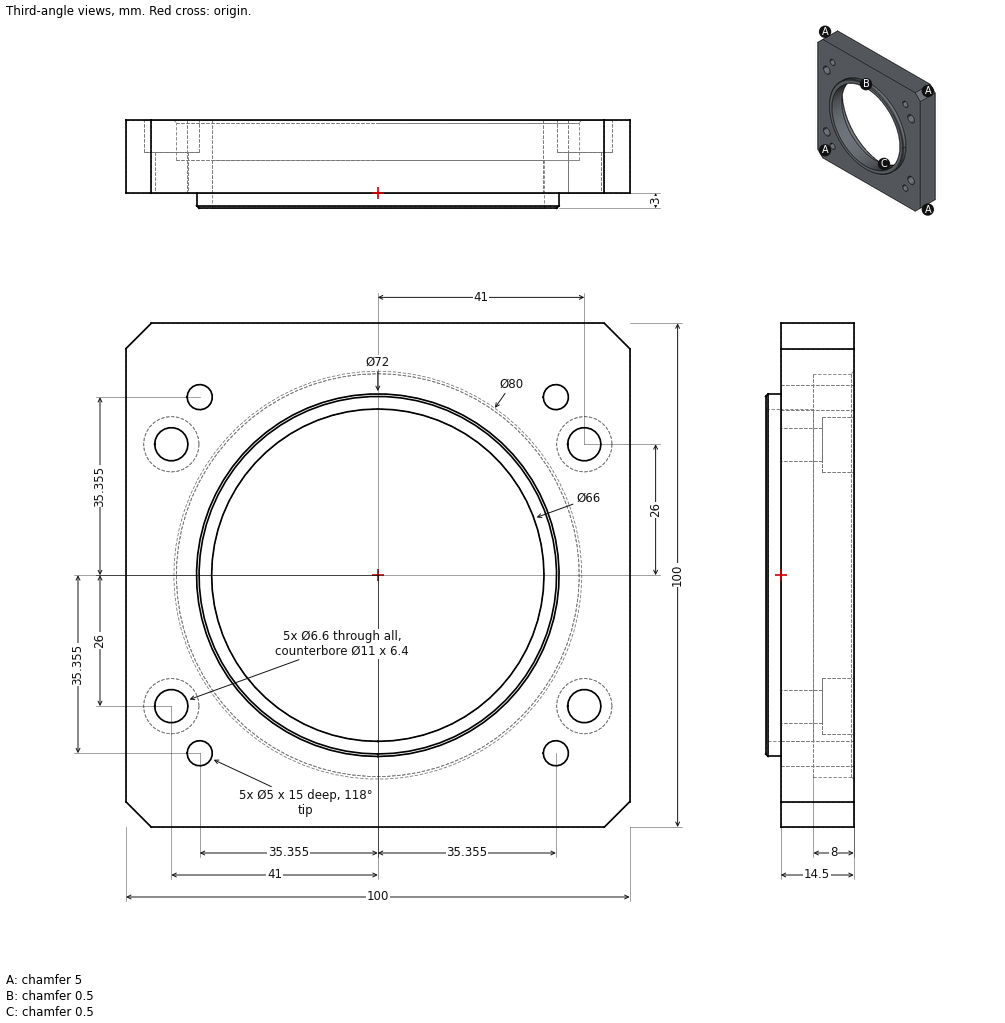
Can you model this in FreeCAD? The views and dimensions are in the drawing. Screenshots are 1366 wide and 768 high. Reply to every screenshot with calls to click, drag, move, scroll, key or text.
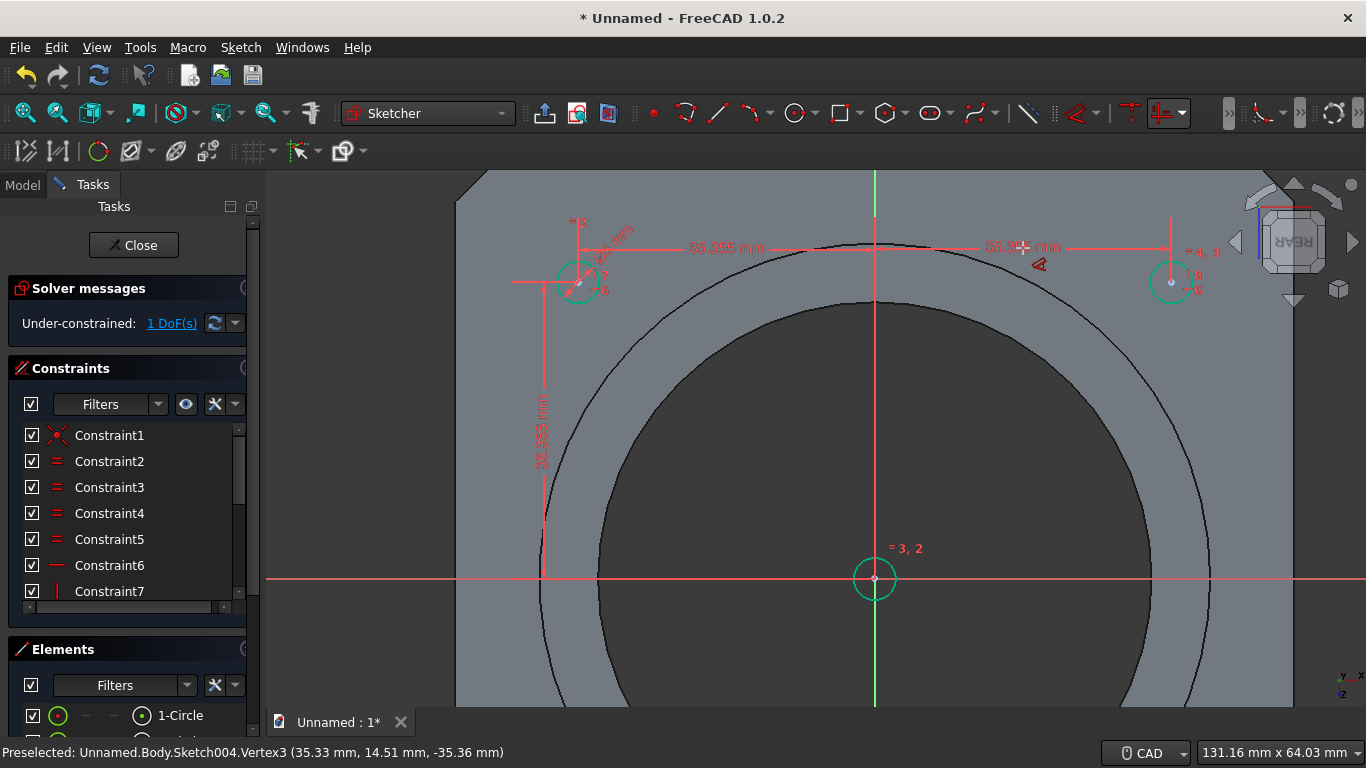
scroll(593, 268, down, 3)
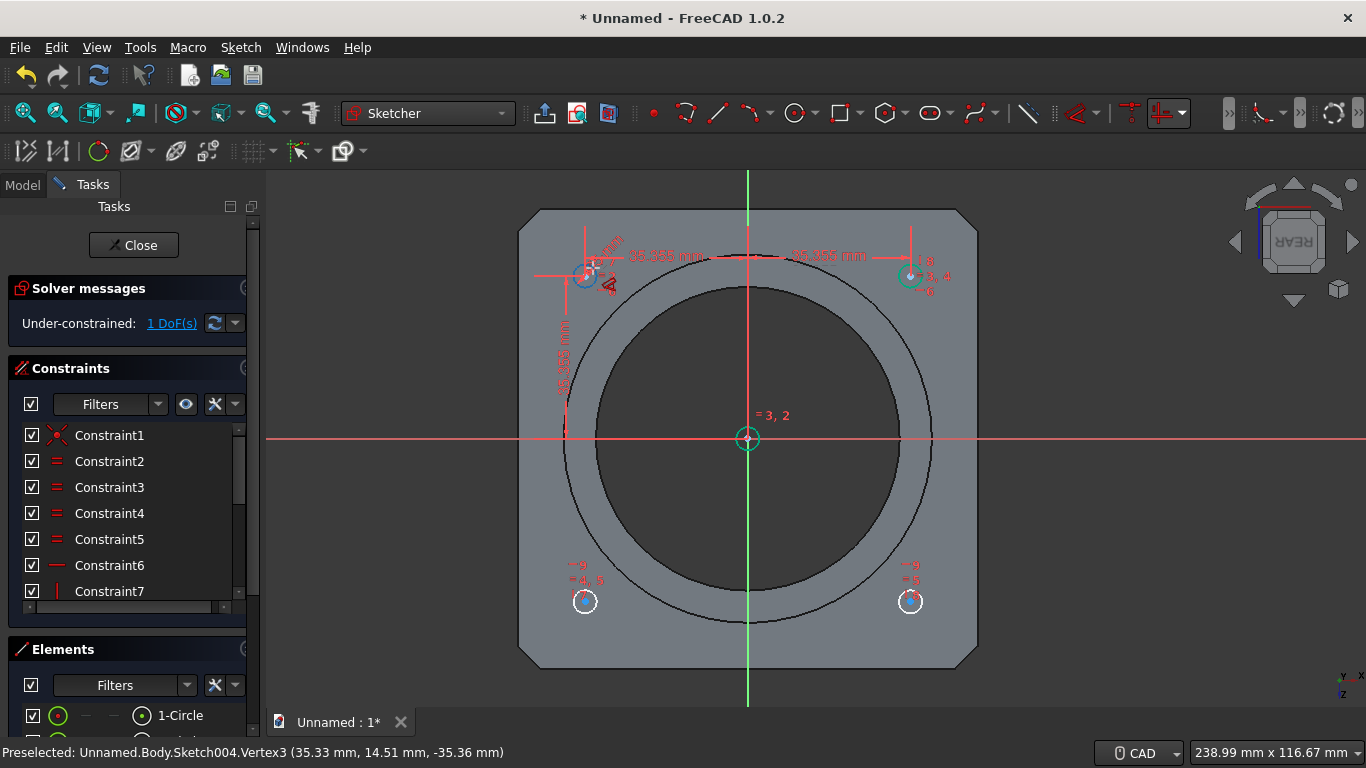
click(585, 602)
click(551, 520)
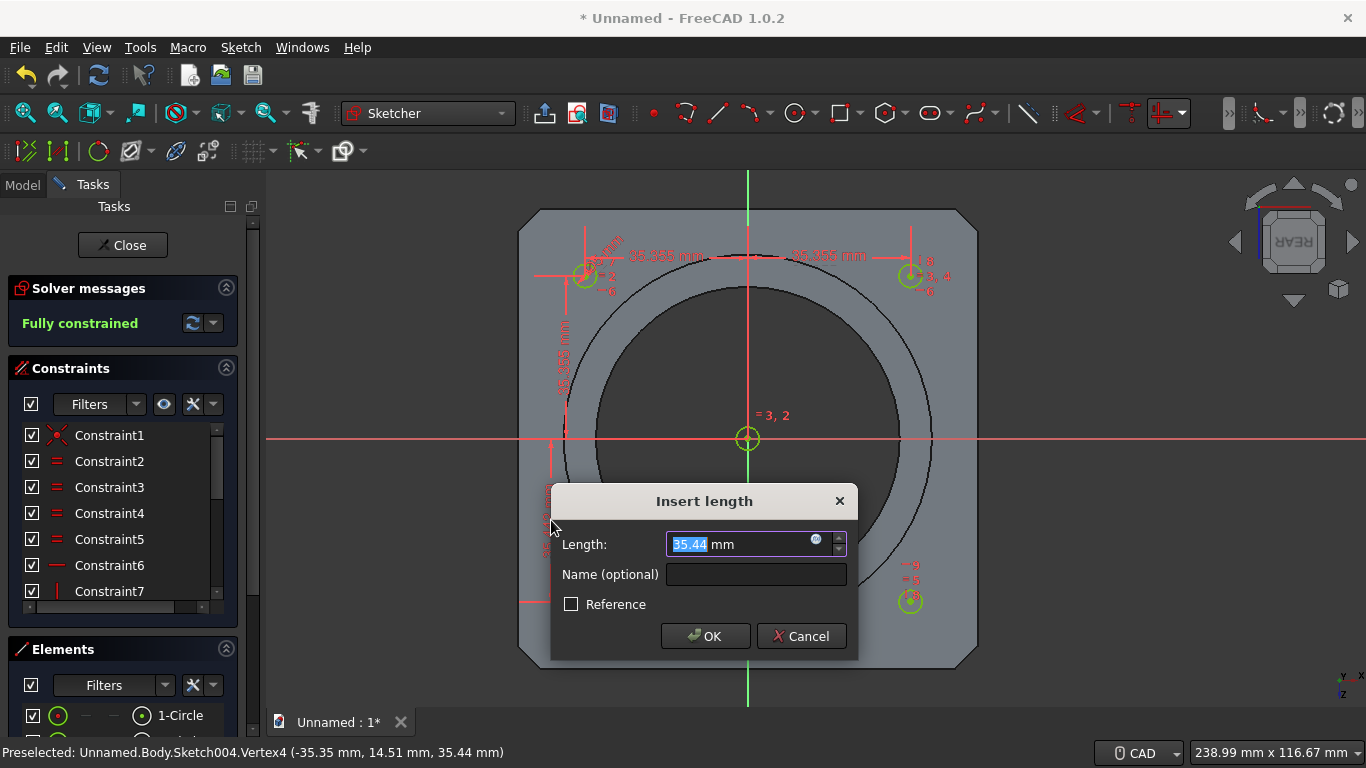
text(35.355)
key(Return)
key(Escape)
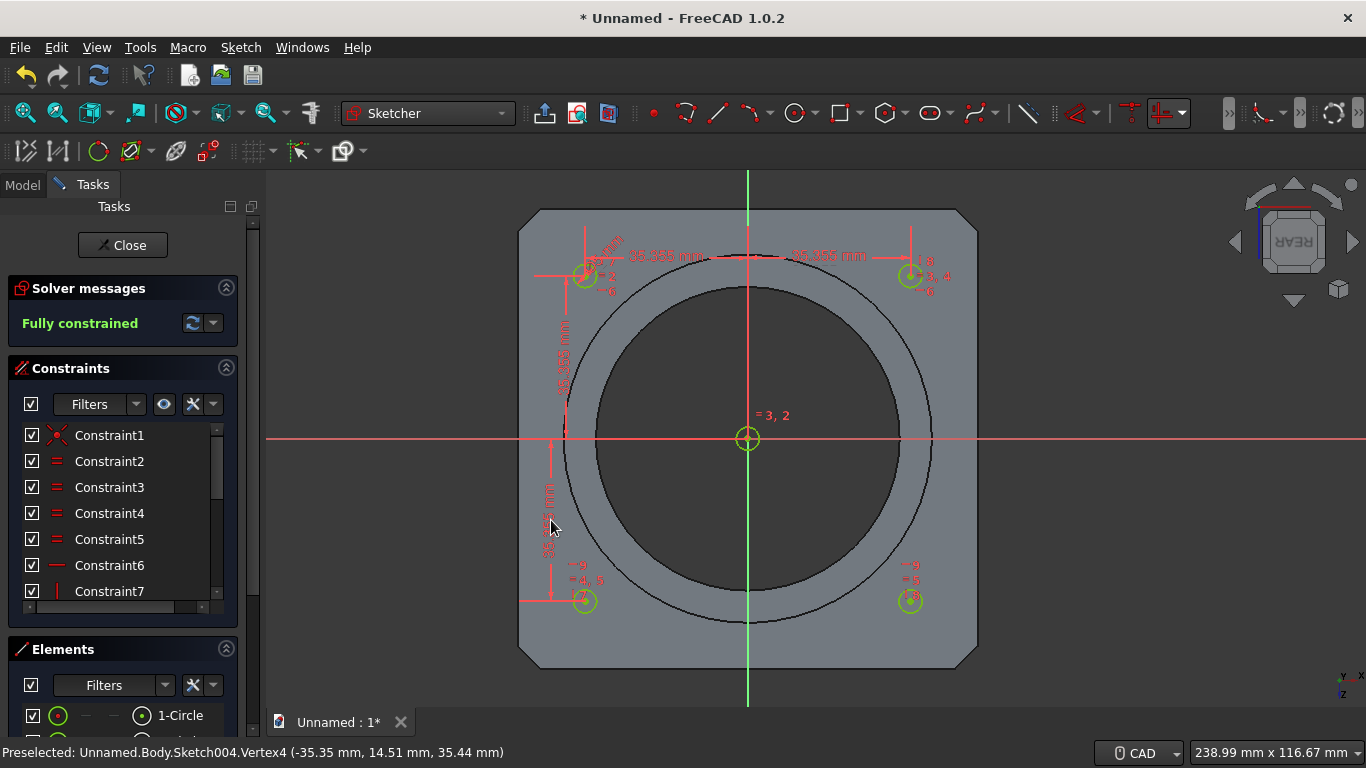
click(123, 245)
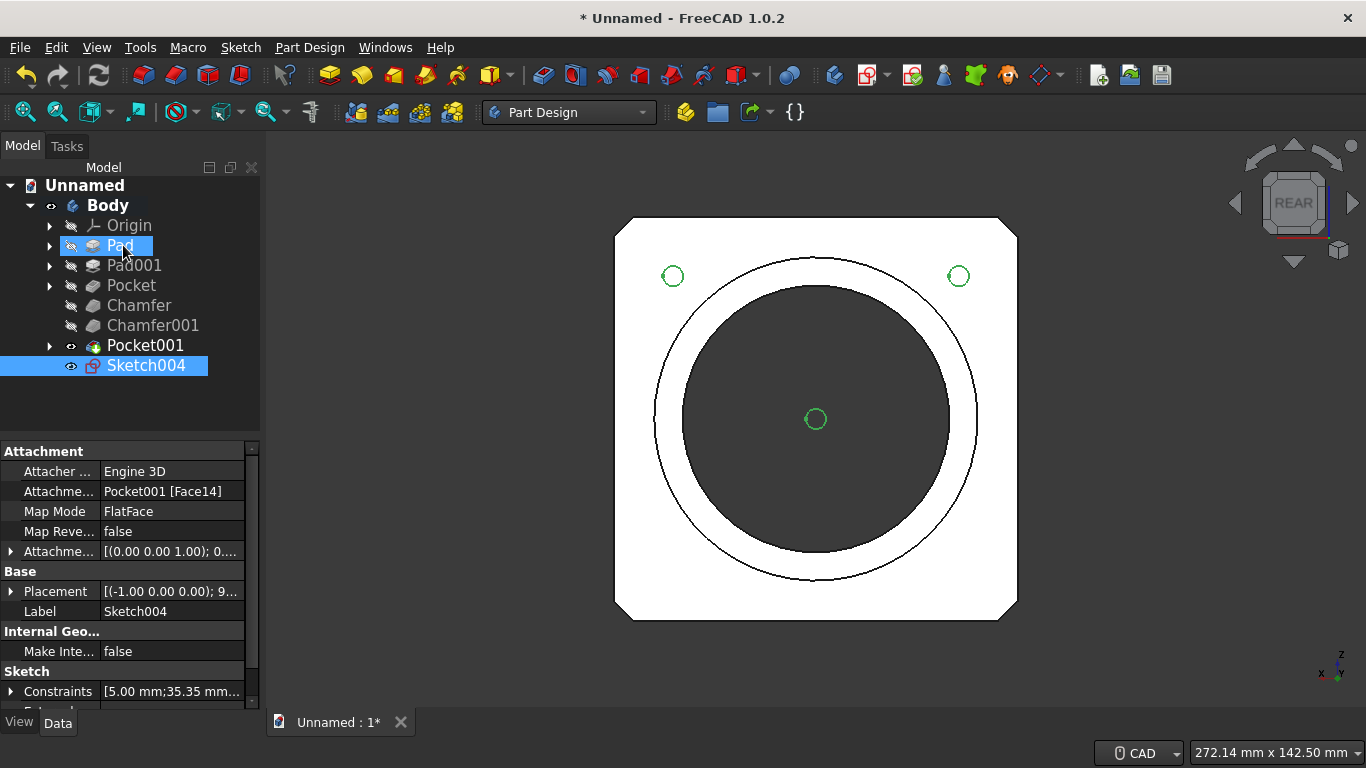
click(576, 76)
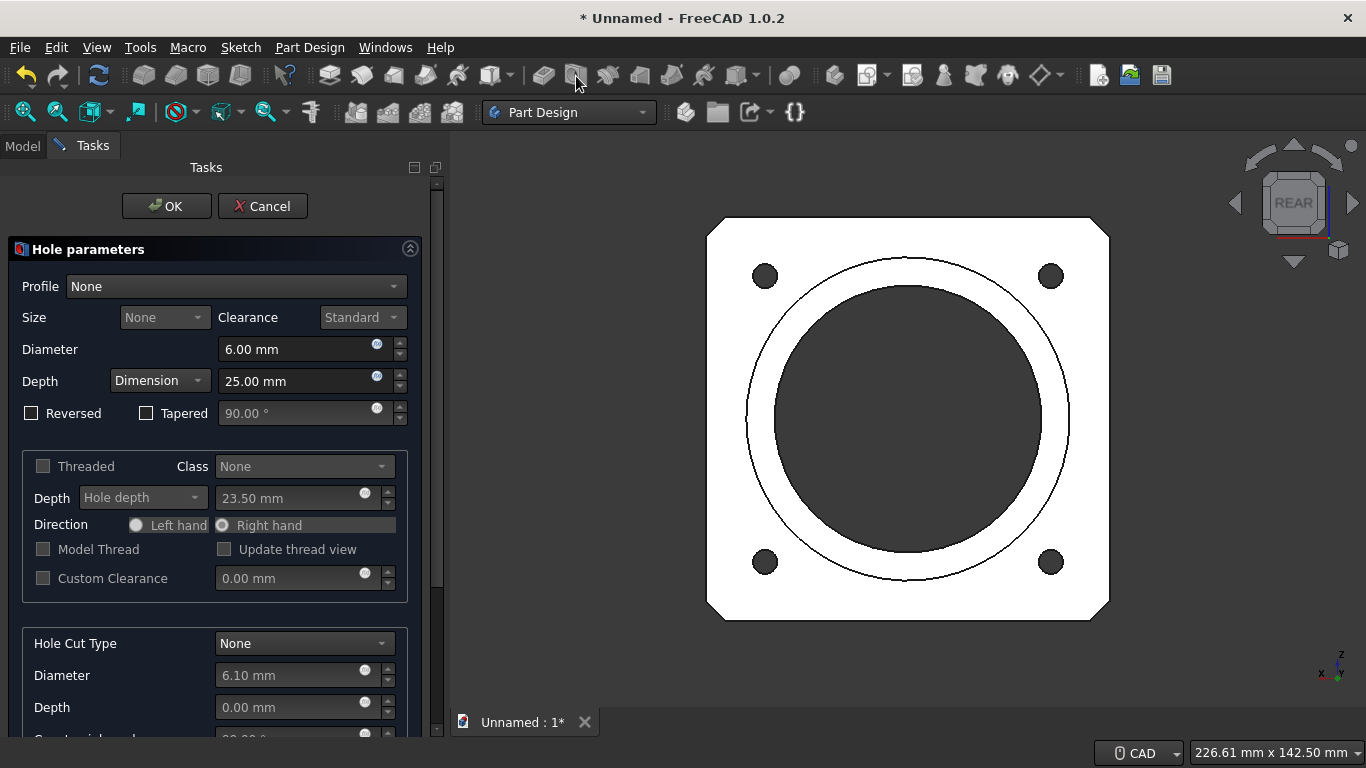
triple_click(305, 349)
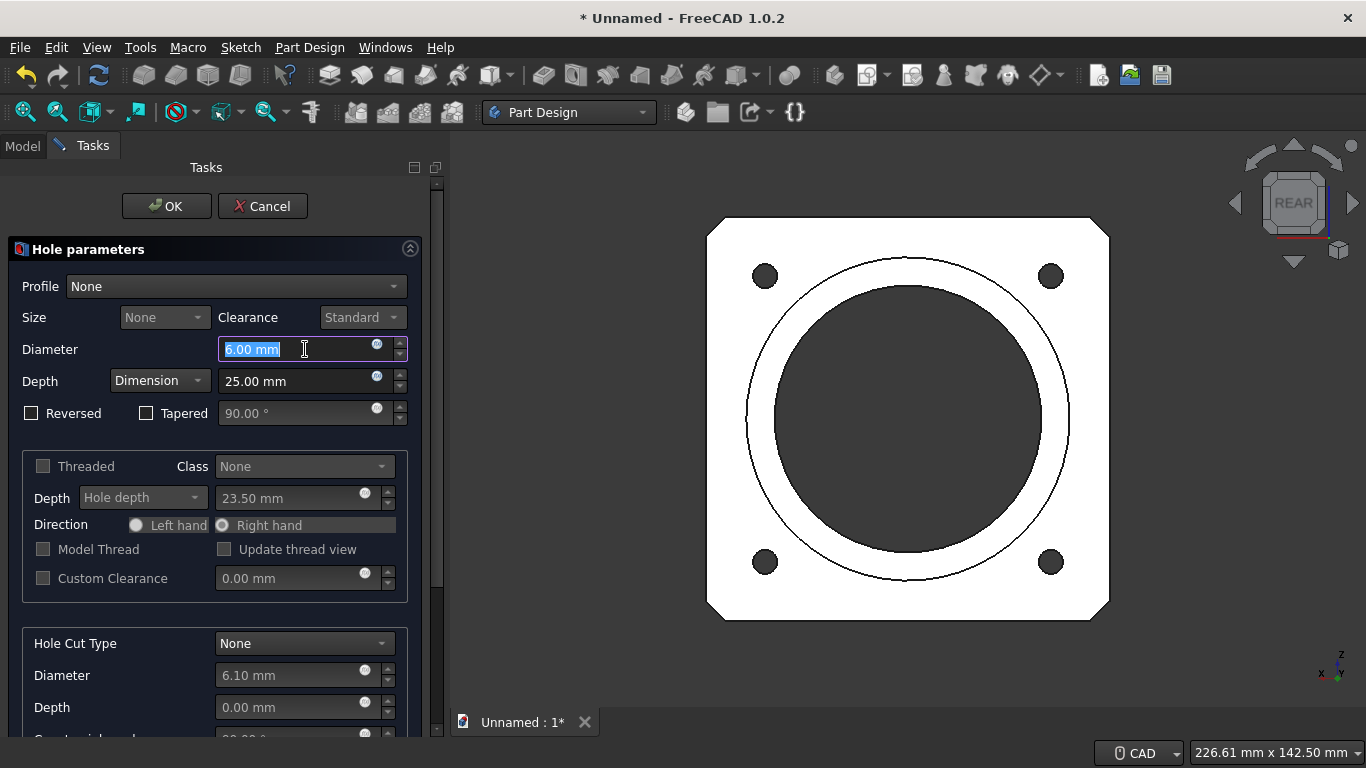
text(5)
key(Tab)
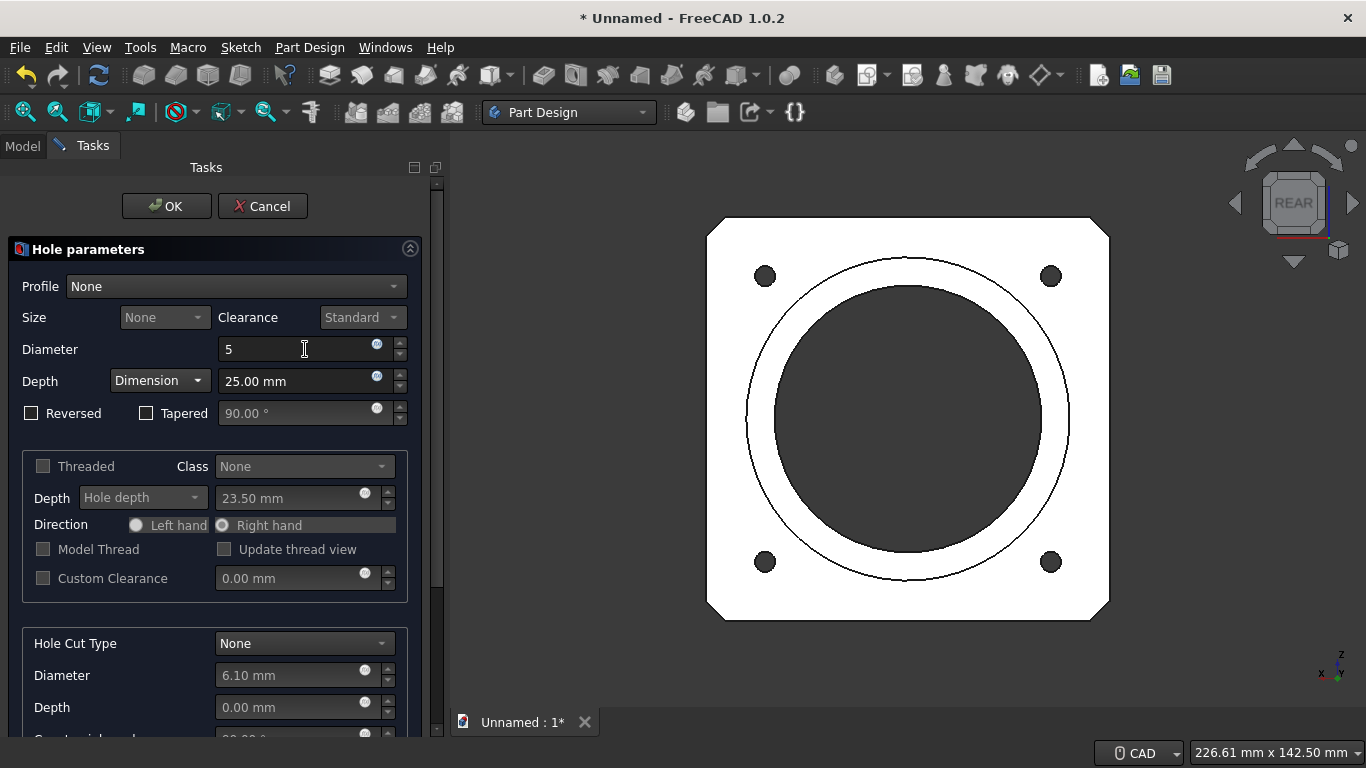
triple_click(305, 381)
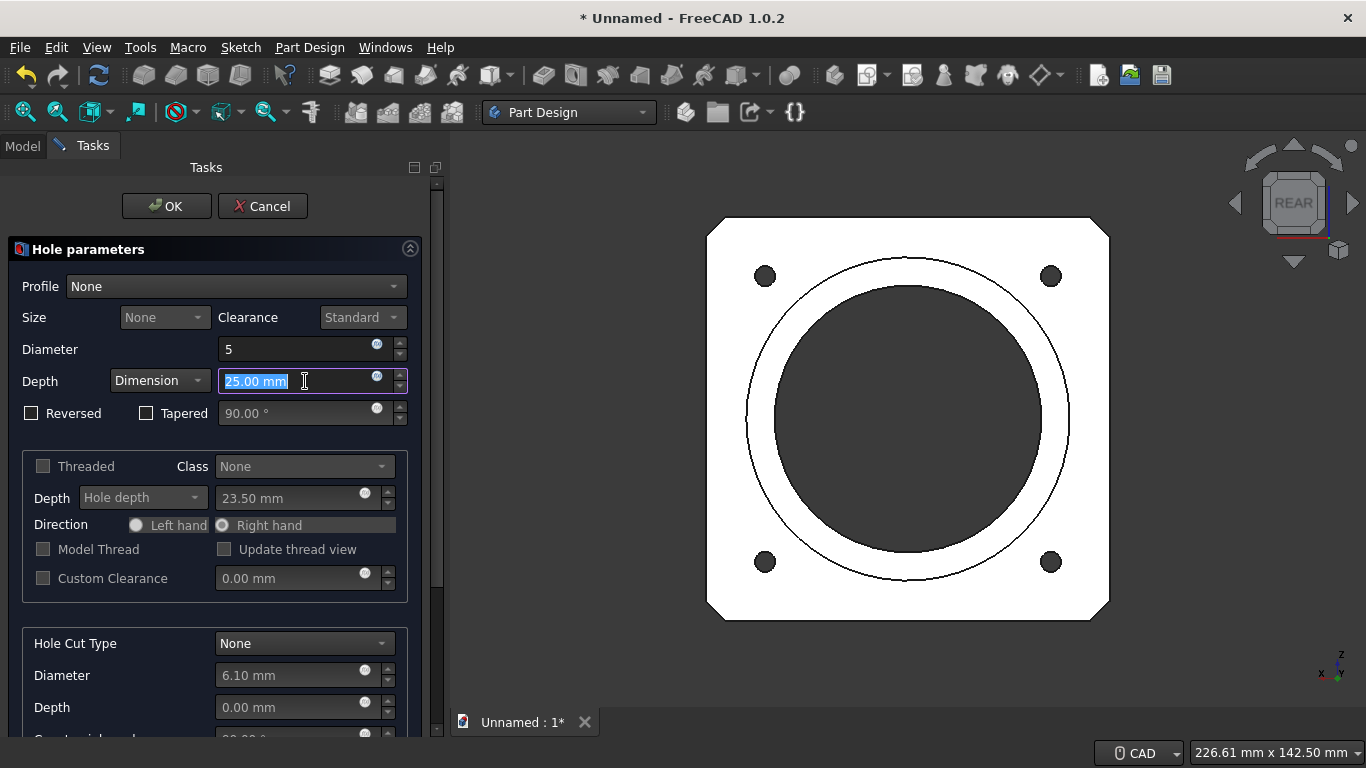
text(15)
key(Tab)